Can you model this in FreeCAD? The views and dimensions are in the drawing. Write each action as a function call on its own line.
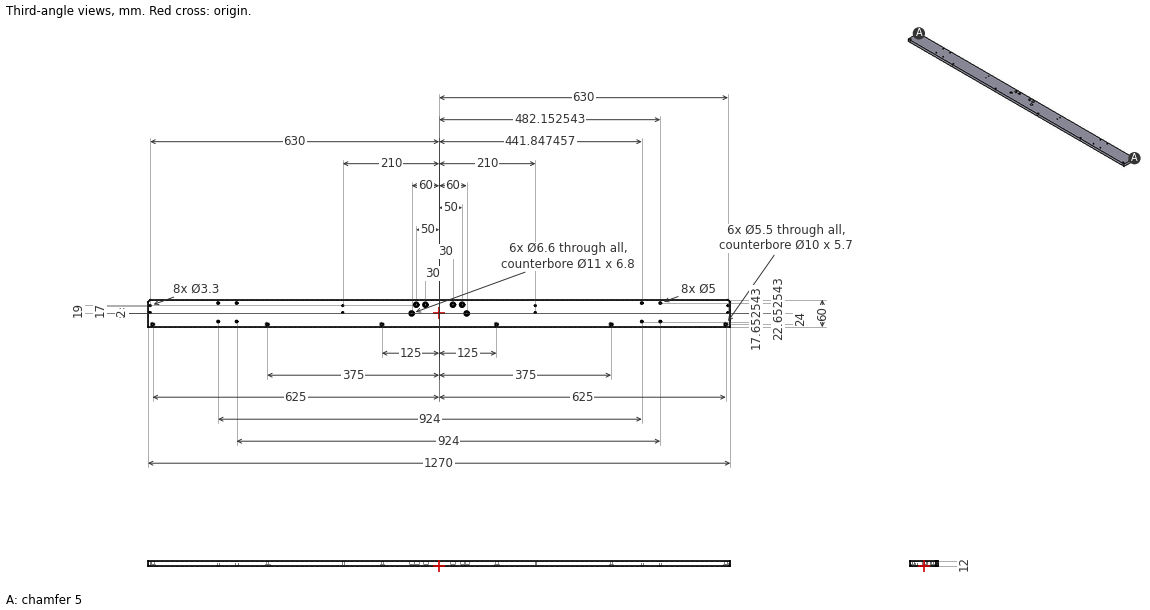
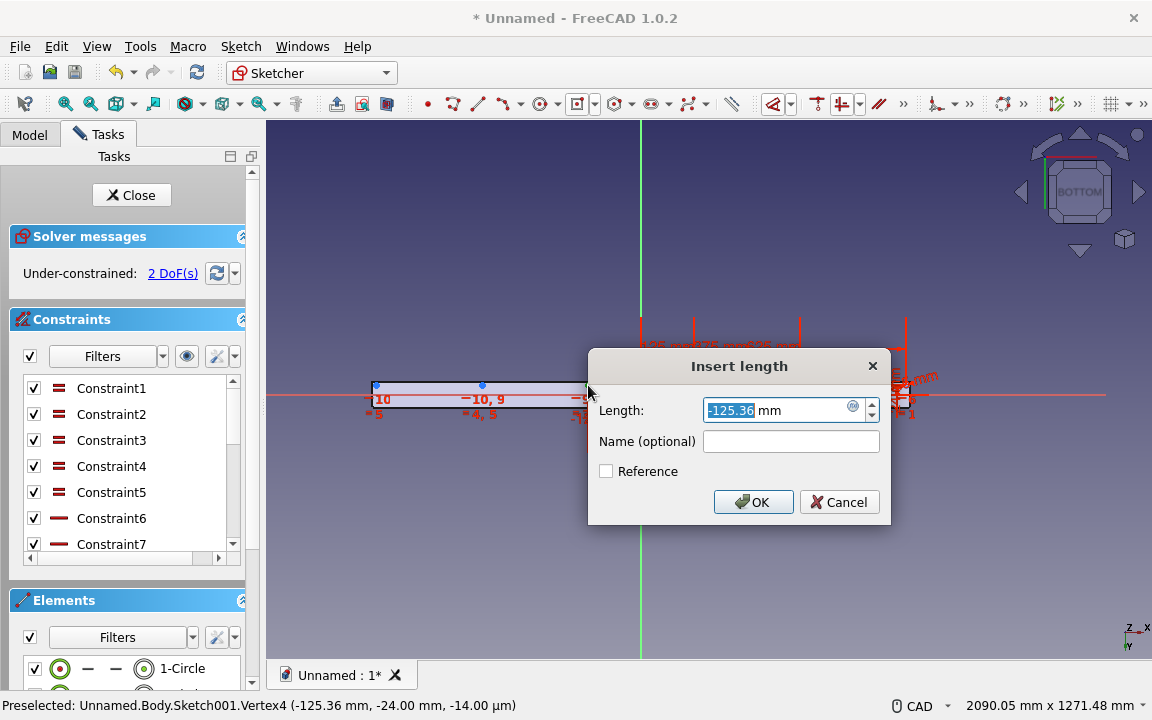
text(-125)
key(Return)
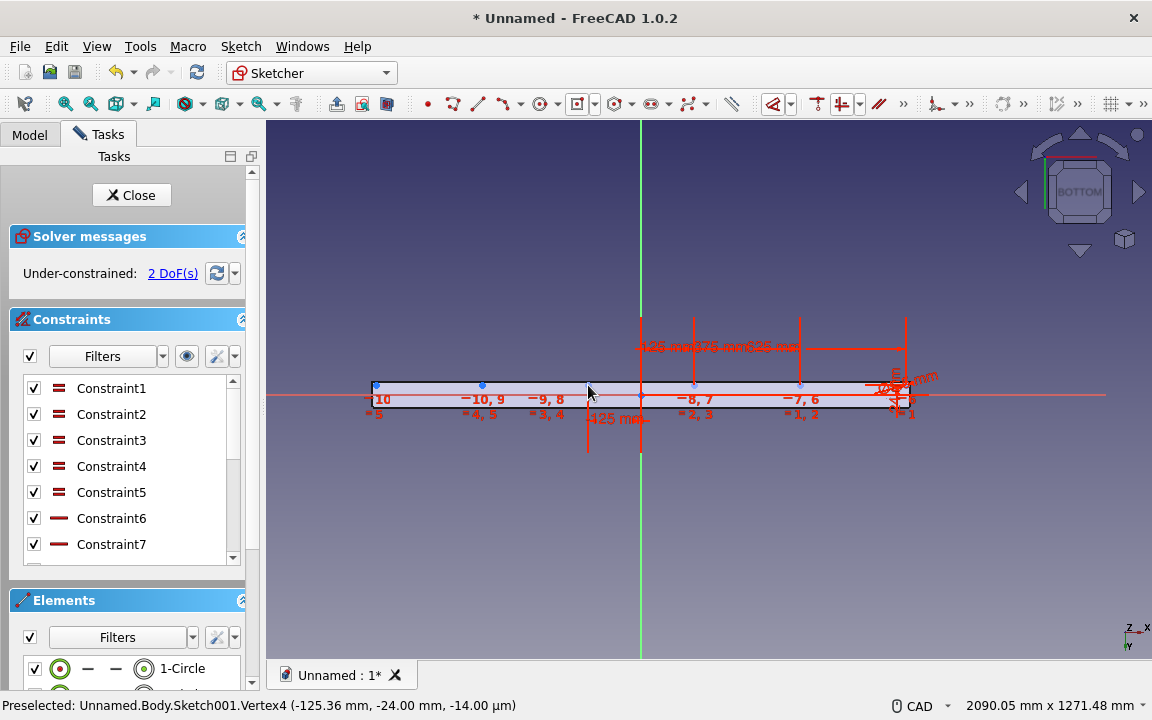
click(482, 385)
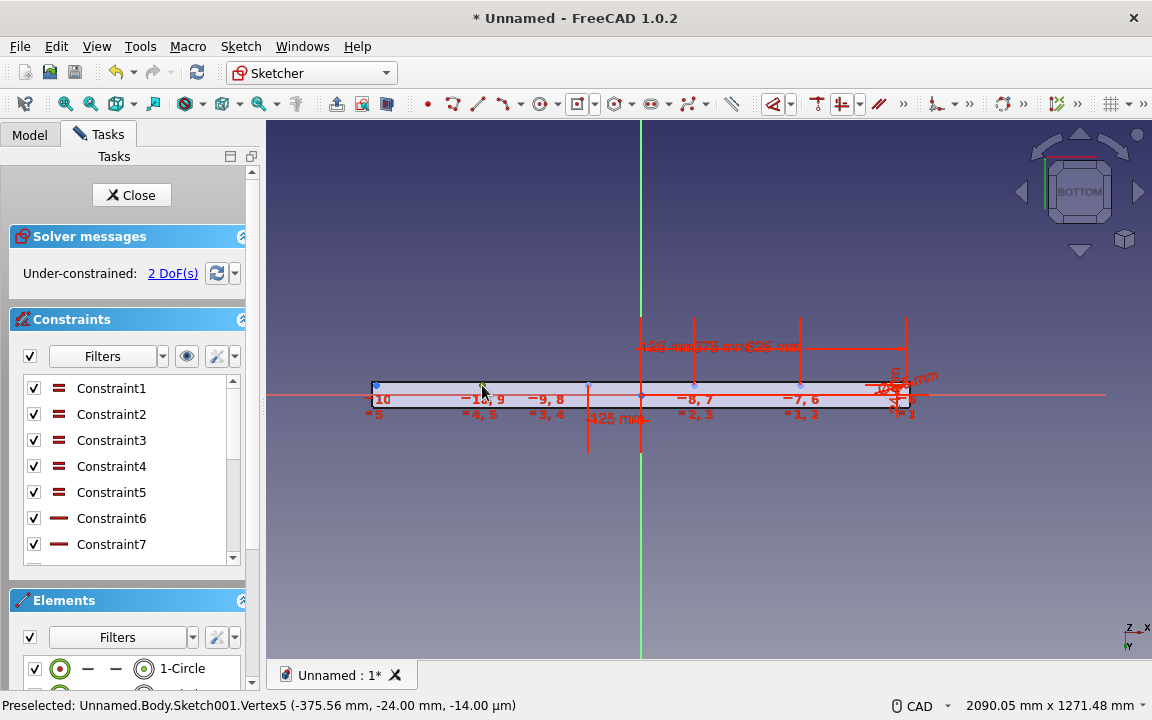
click(790, 104)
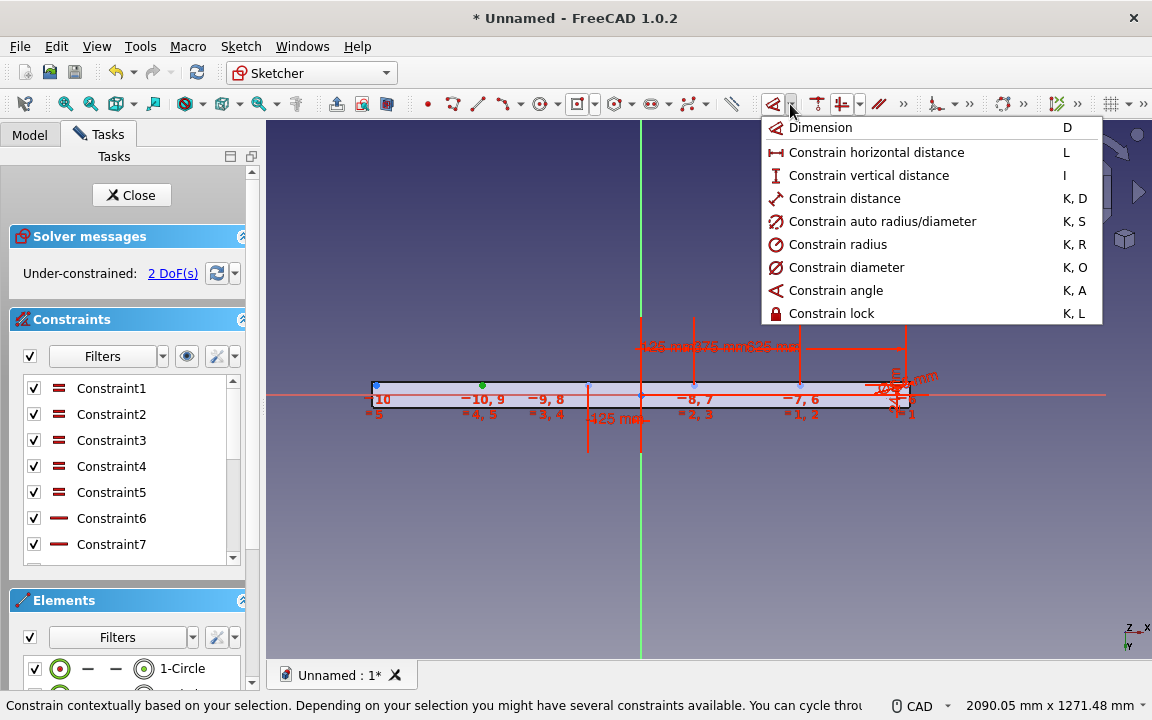
click(932, 152)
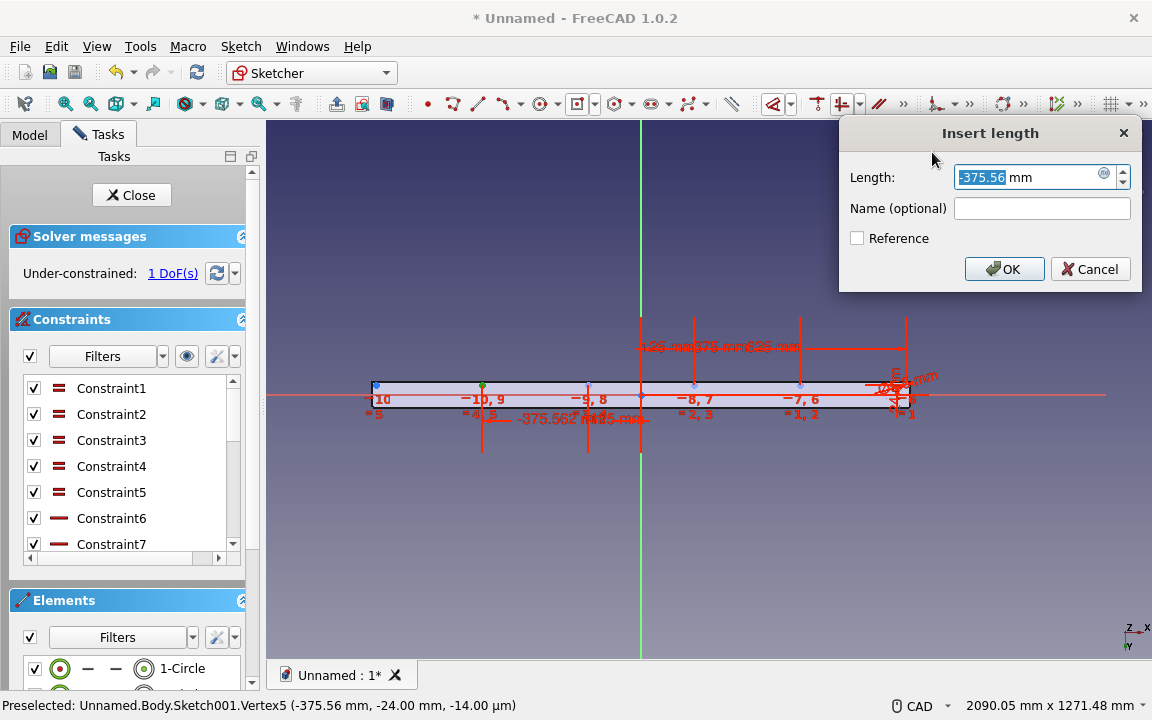
text(-375)
key(Return)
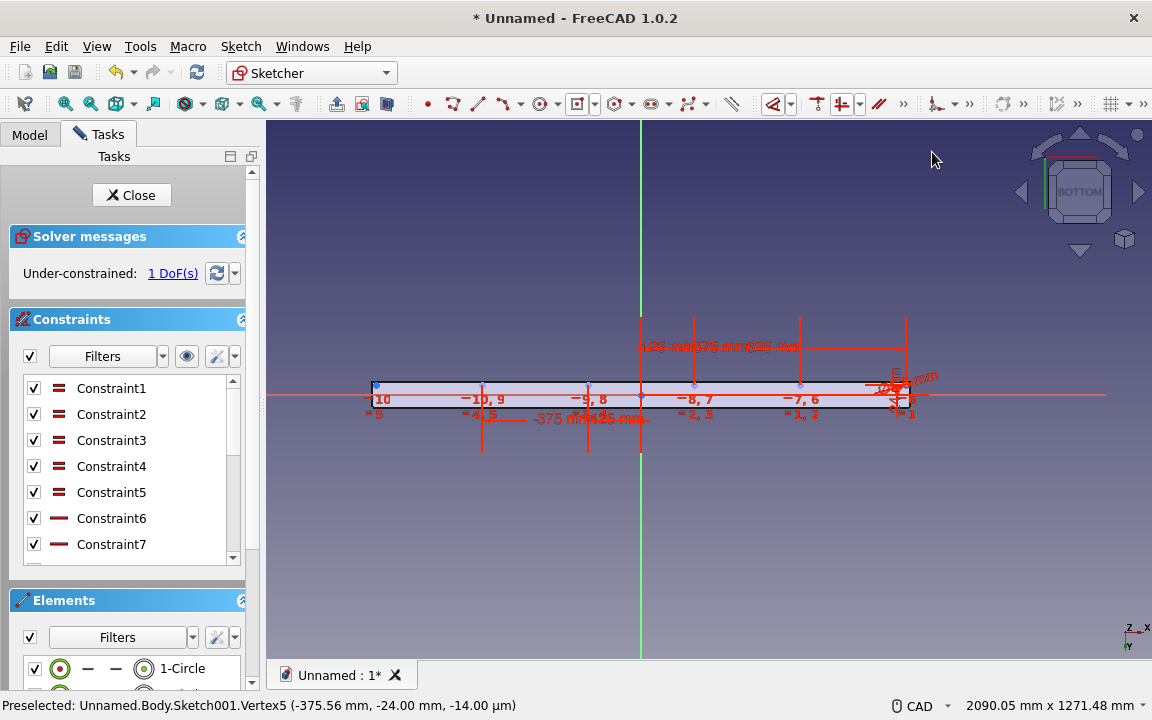
click(377, 385)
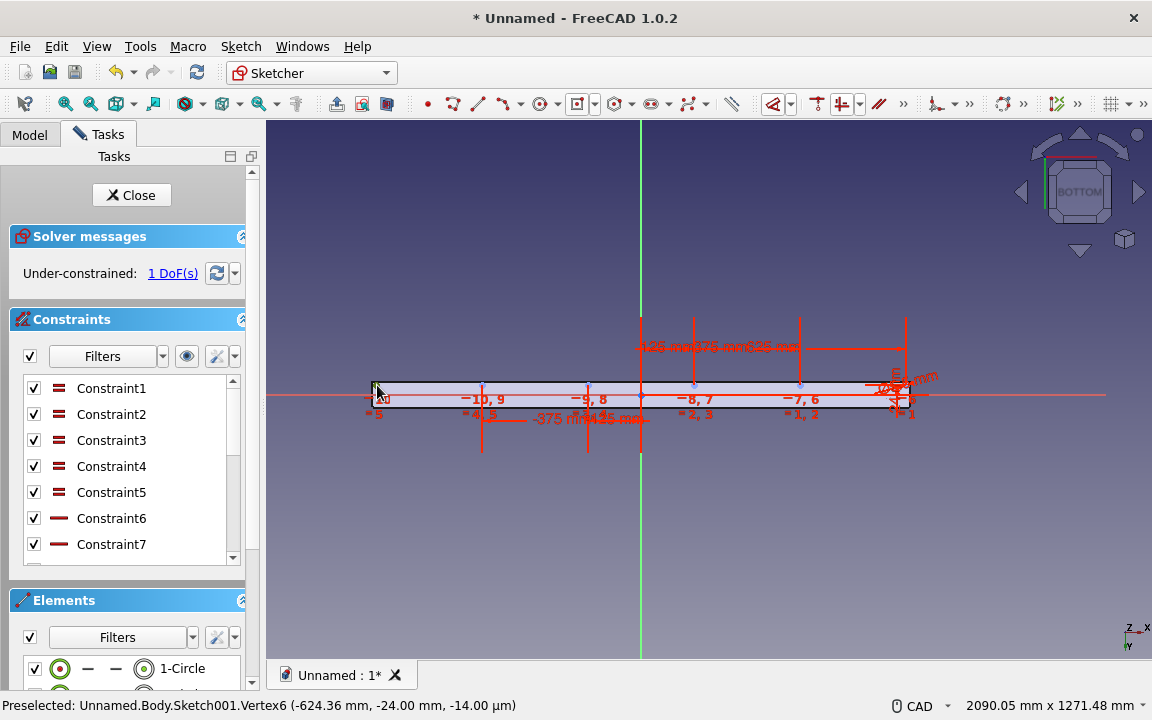
key(l)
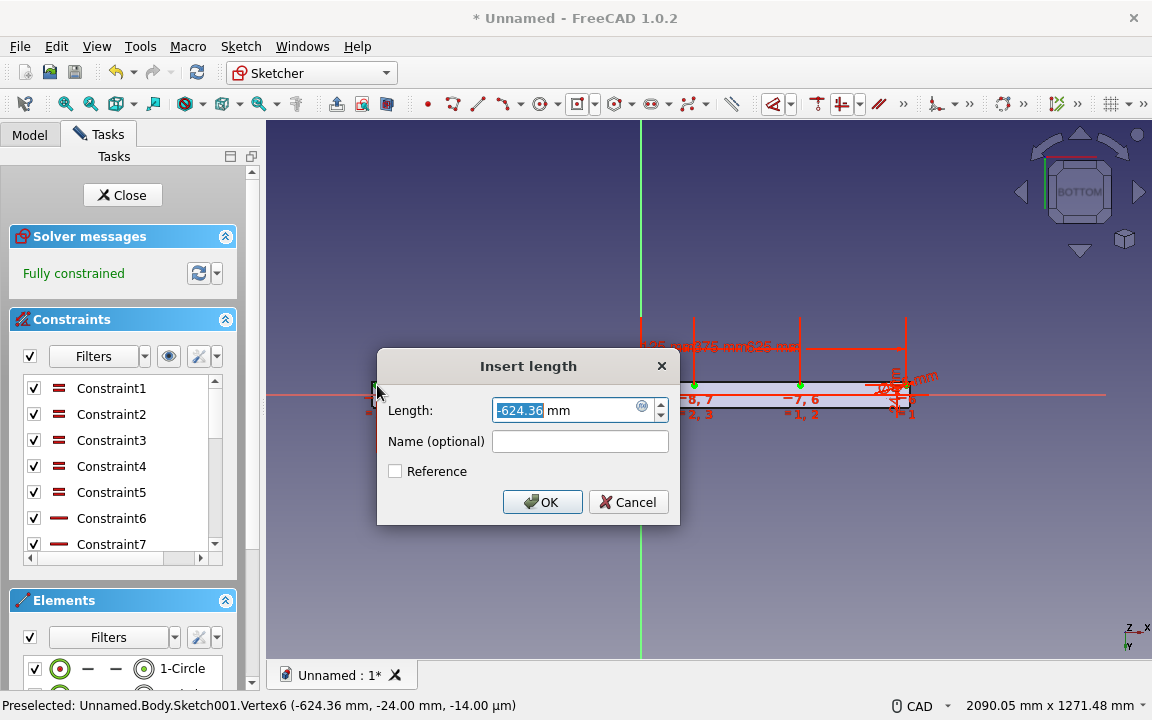
text(-625)
key(Return)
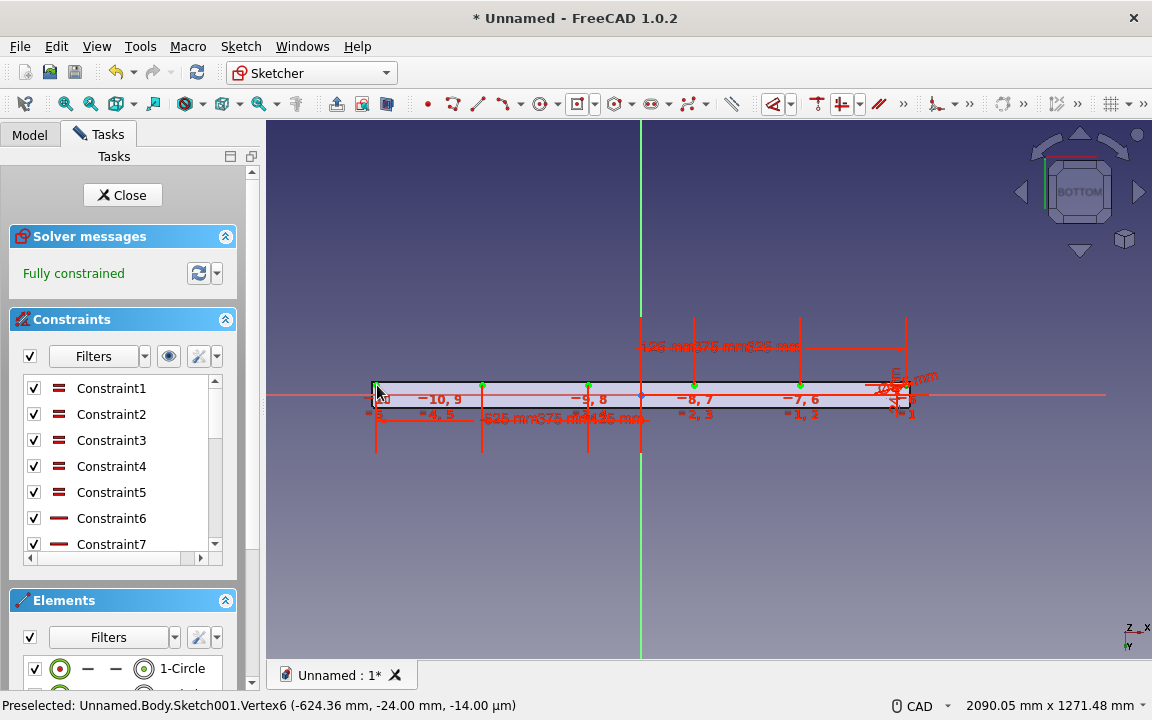
click(123, 195)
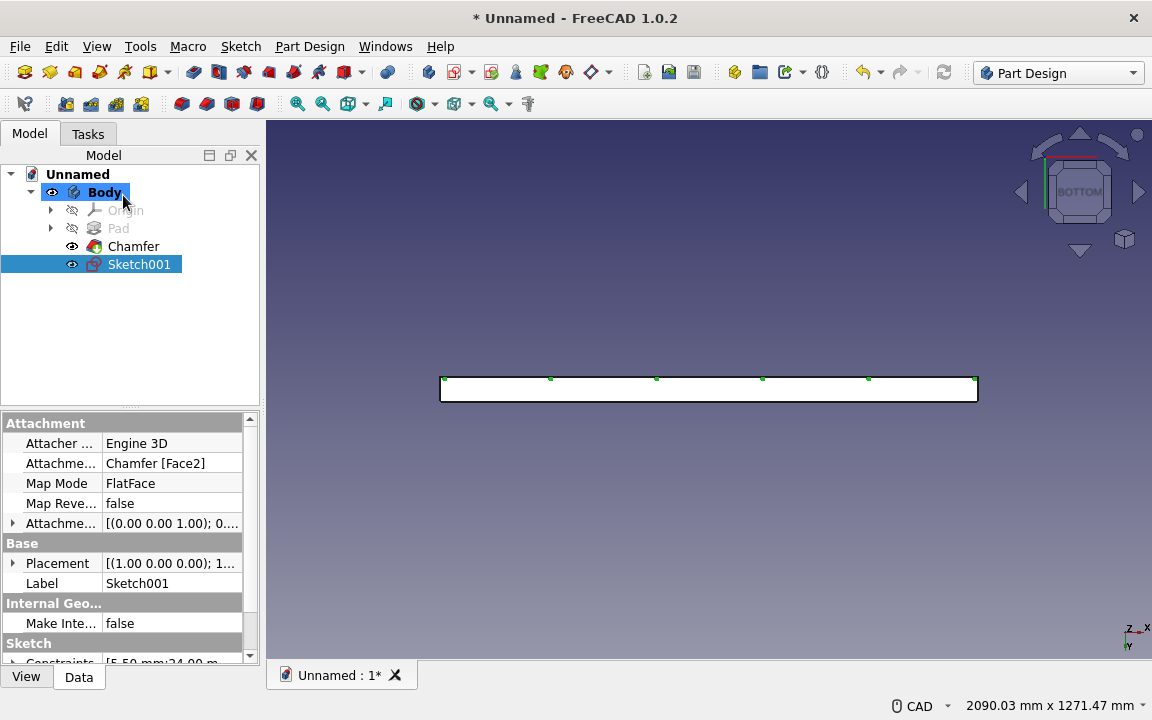
click(219, 72)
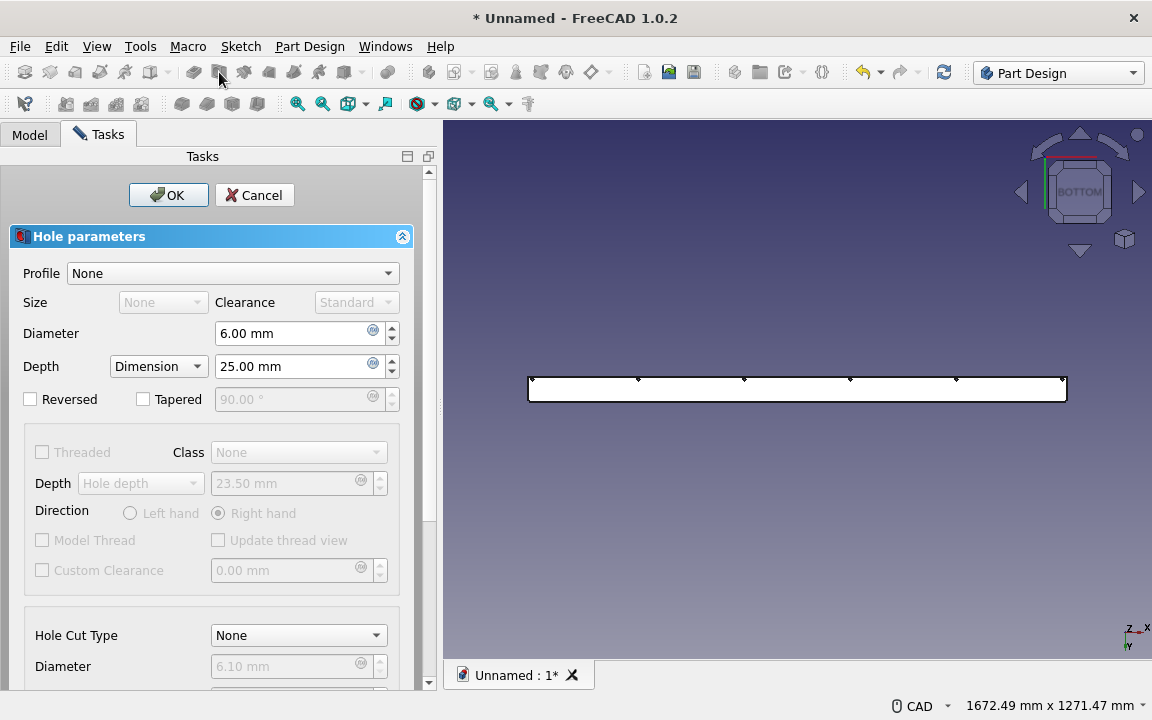
triple_click(300, 334)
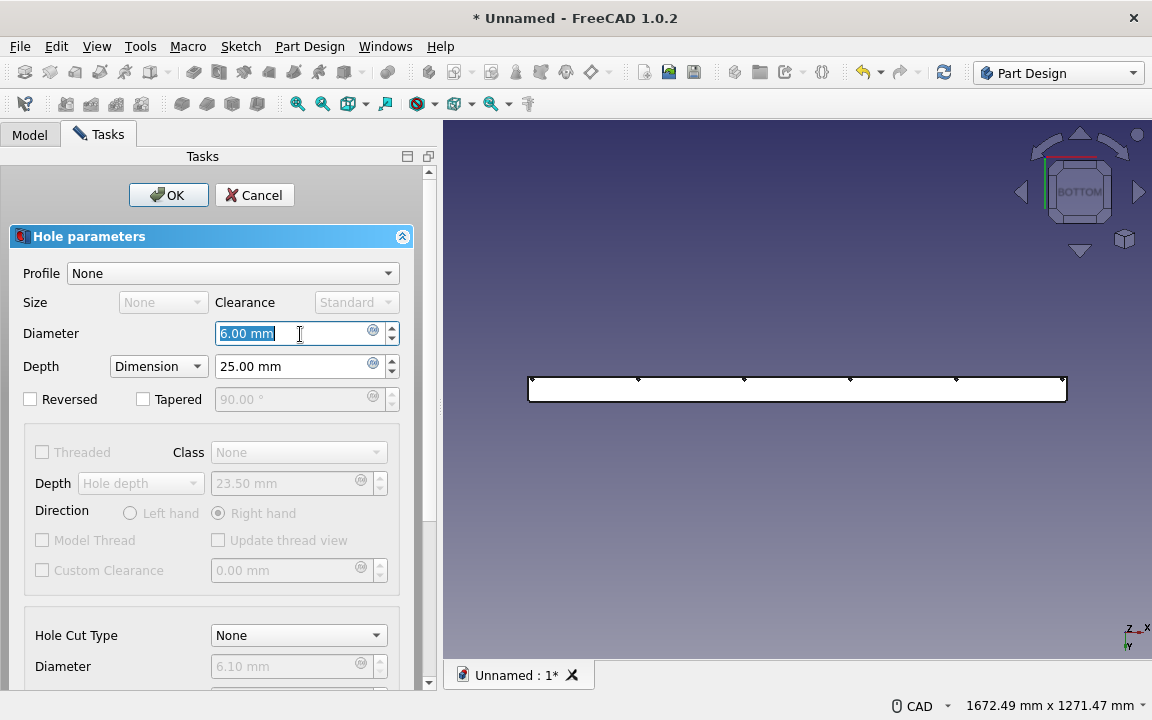
text(5.5)
key(Tab)